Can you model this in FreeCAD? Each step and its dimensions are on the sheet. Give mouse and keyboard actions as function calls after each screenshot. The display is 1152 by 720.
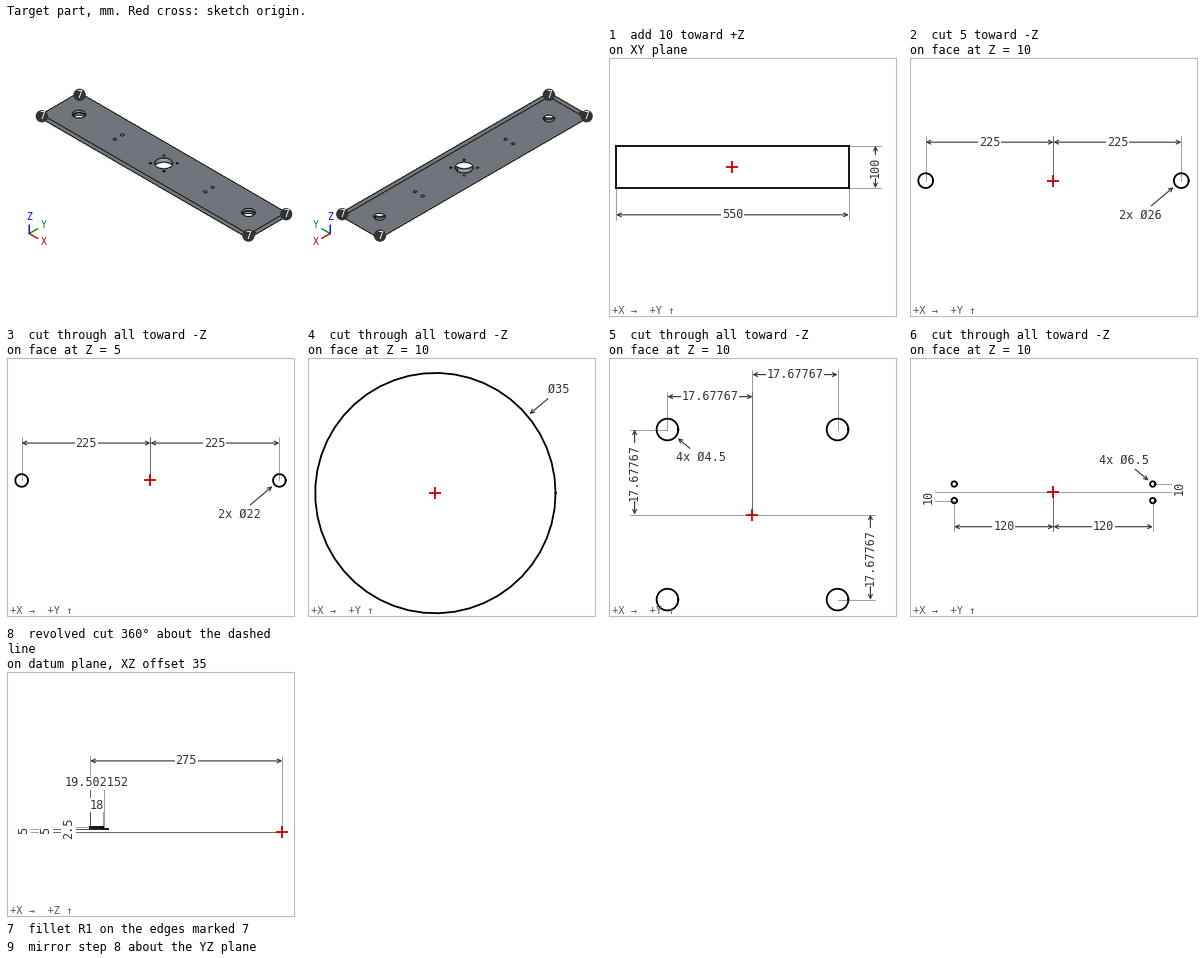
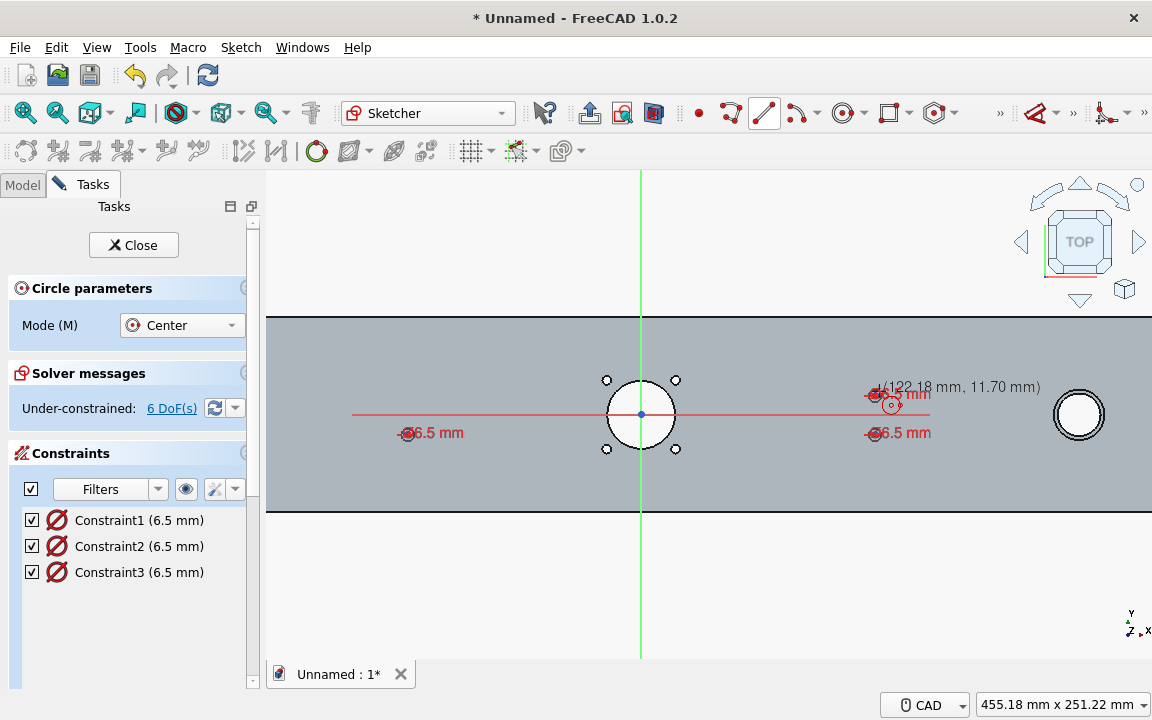
scroll(408, 395, up, 7)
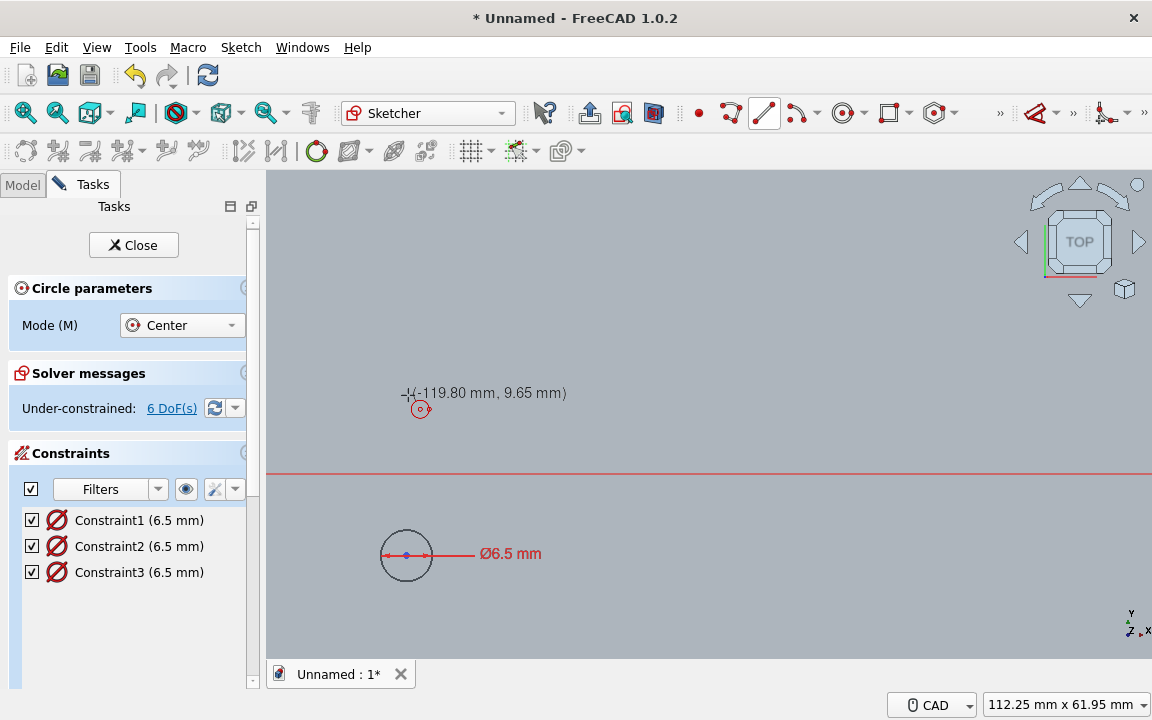
scroll(407, 395, down, 7)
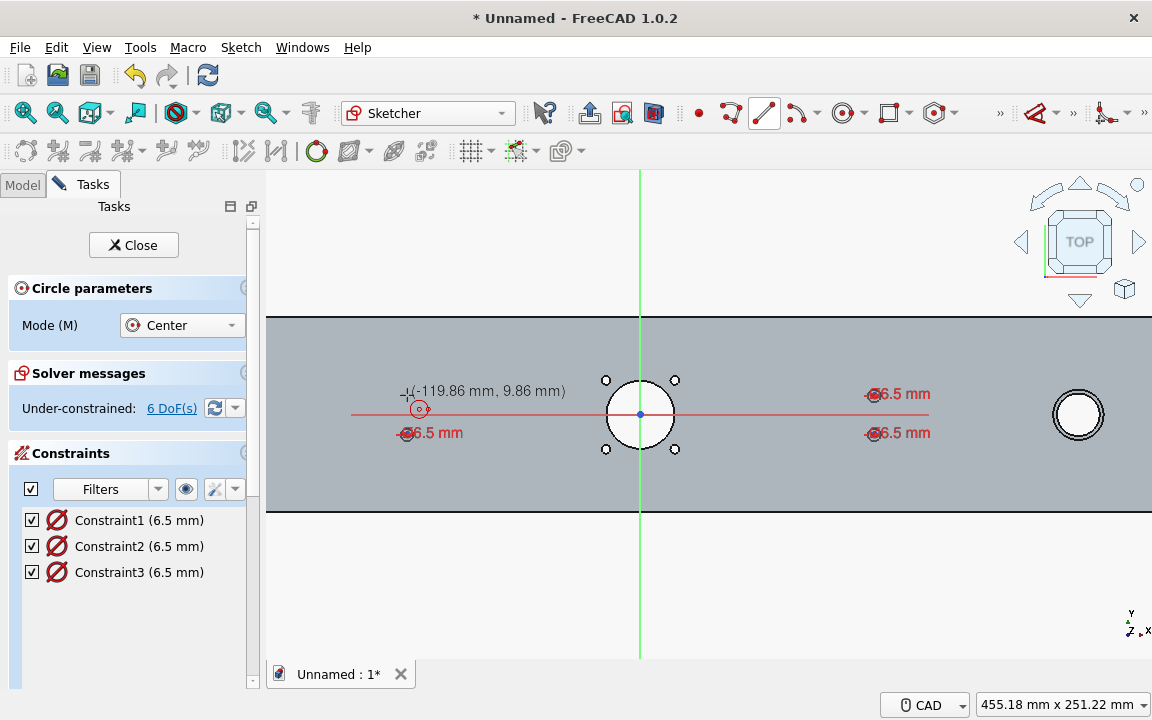
click(407, 395)
move(411, 391)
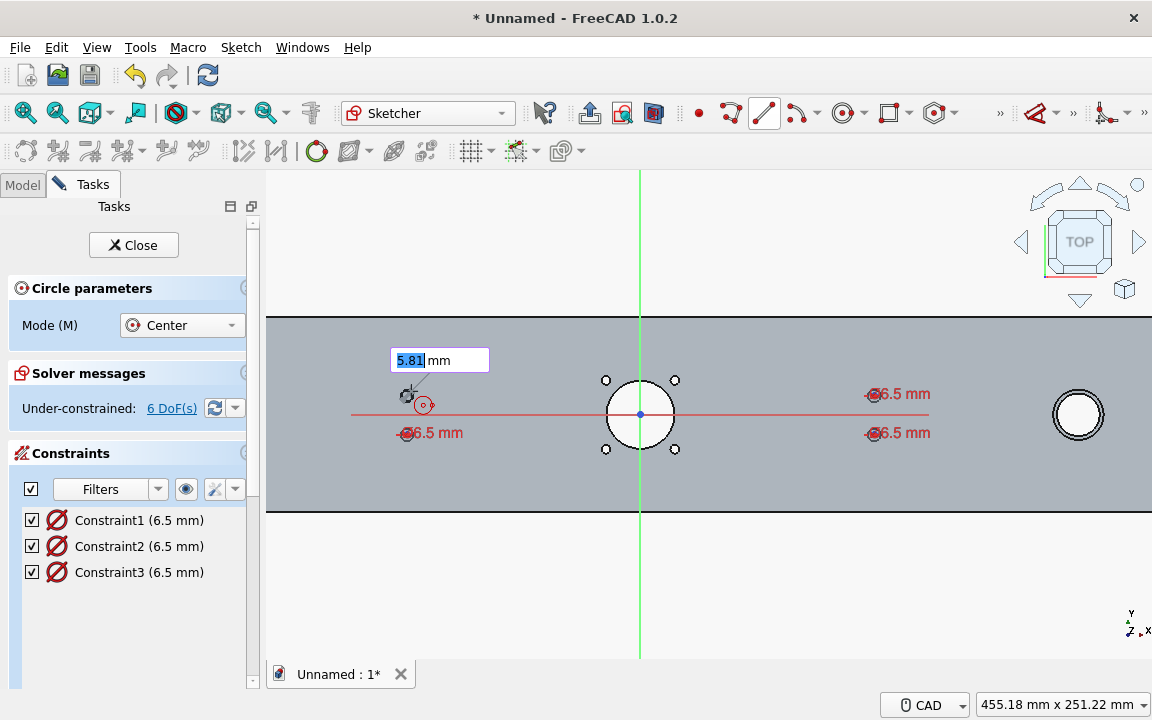
text(6.5)
key(Return)
key(Escape)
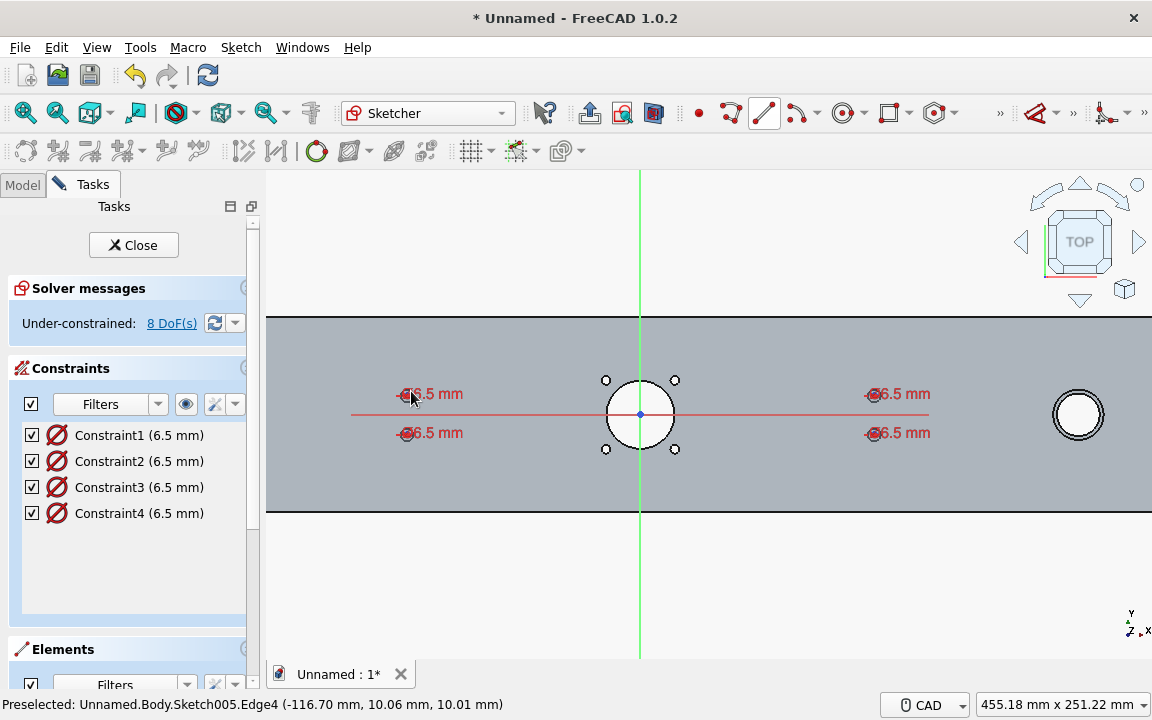
click(407, 435)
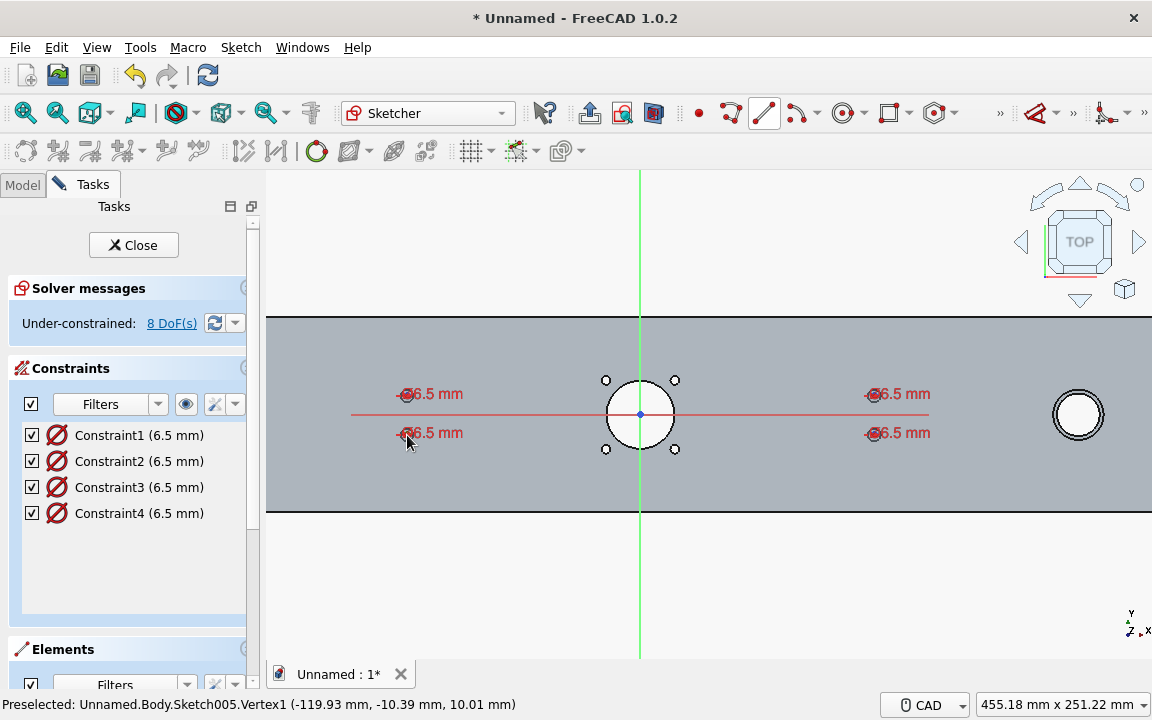
click(874, 435)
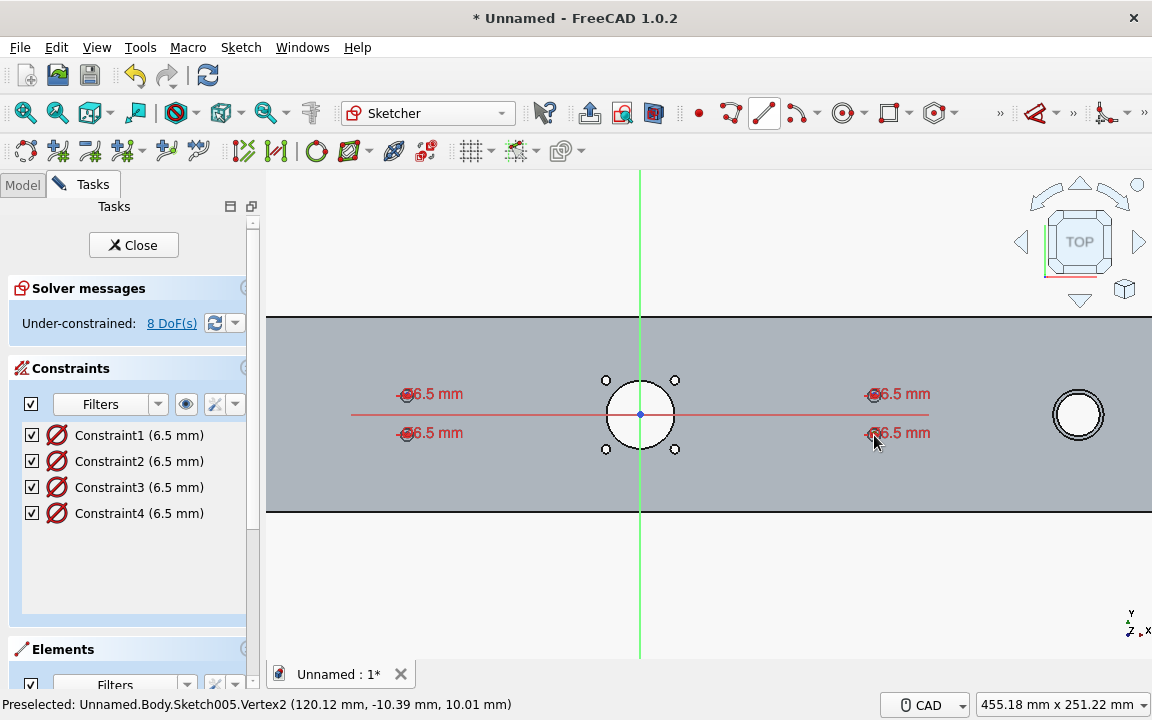
key(h)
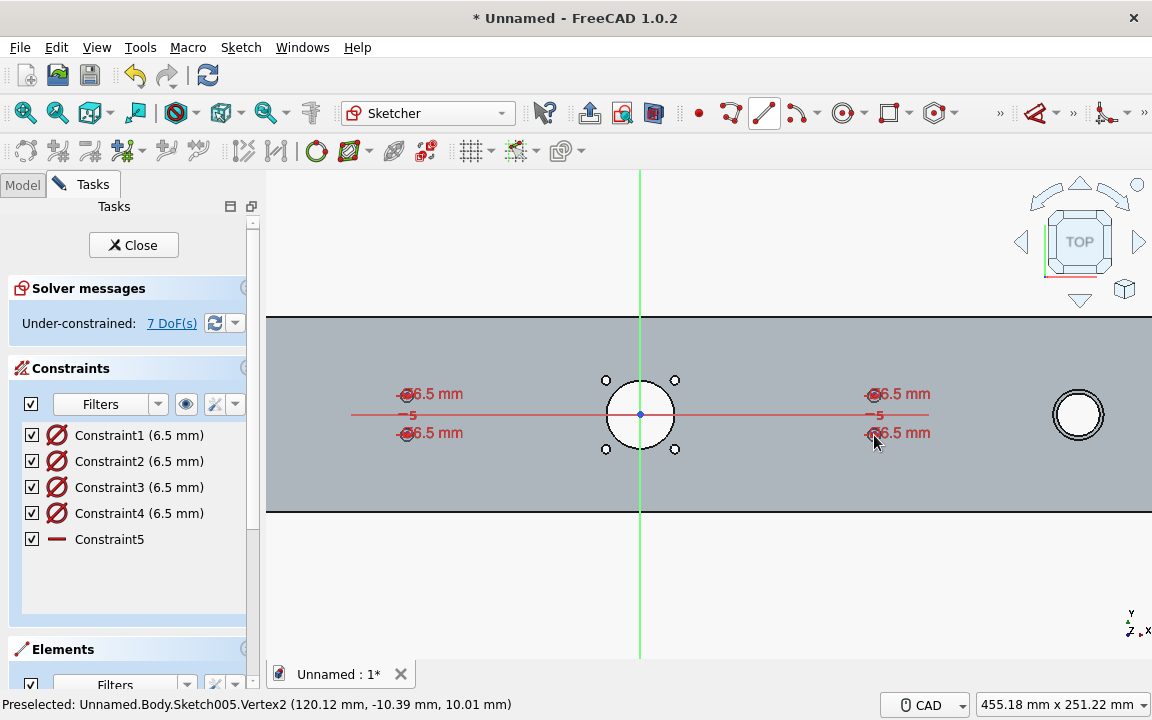
click(874, 435)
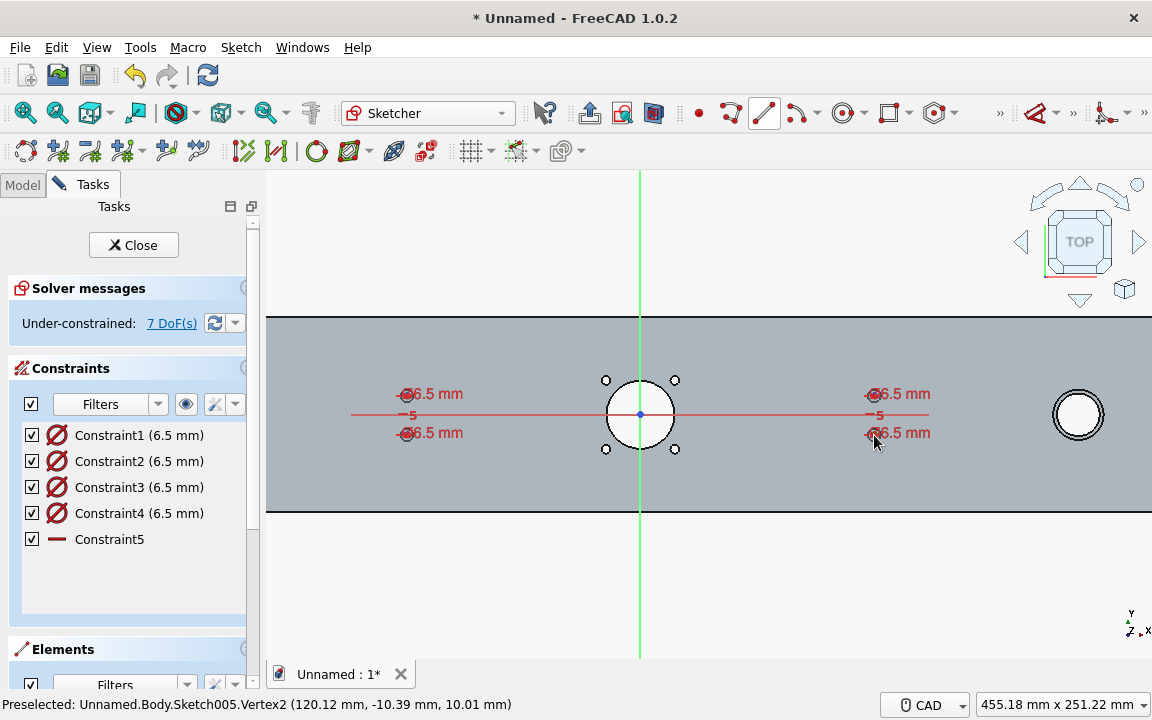
click(874, 396)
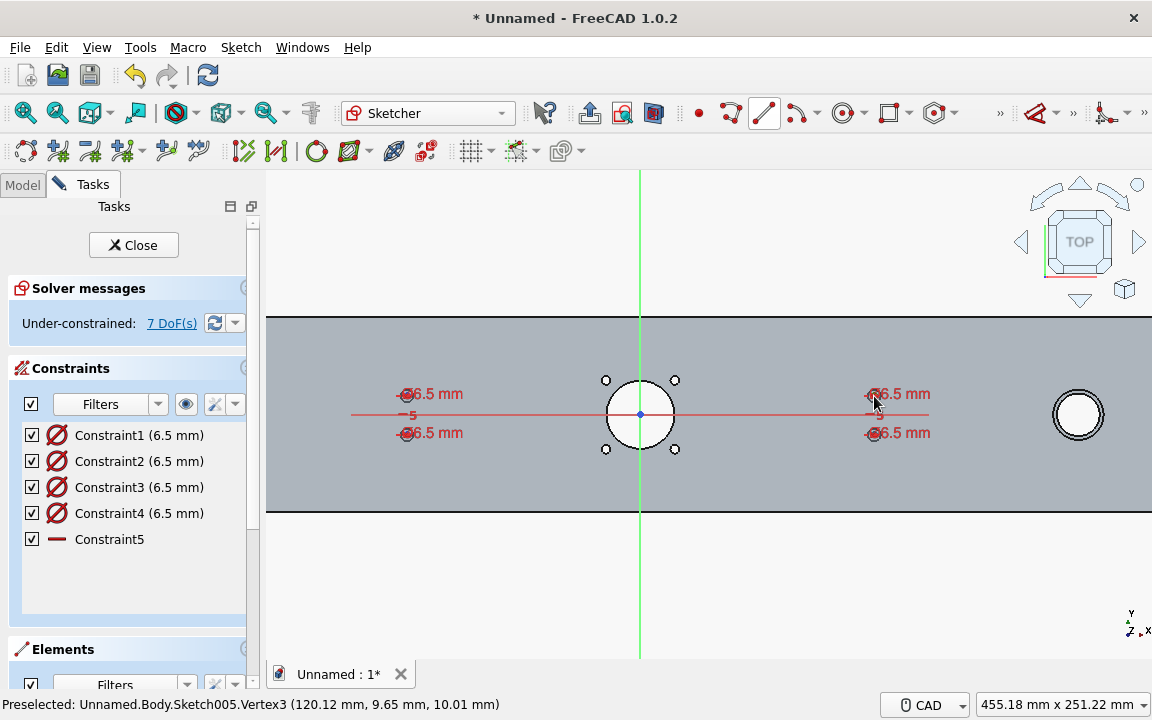
key(v)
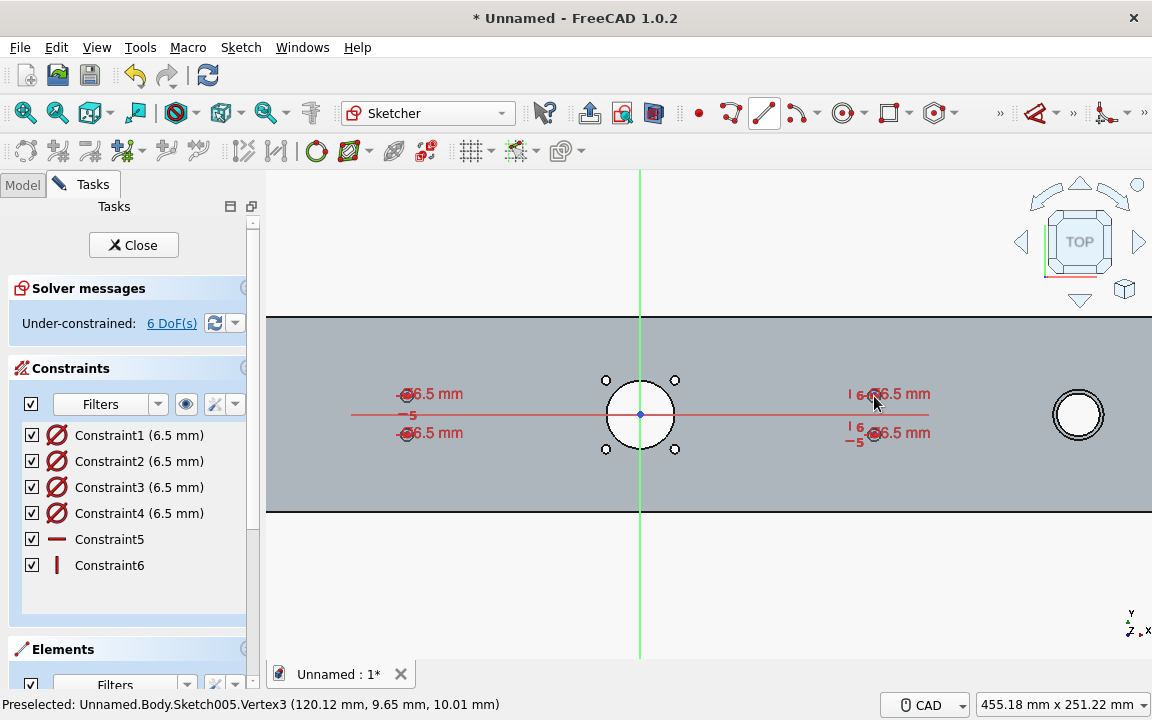
click(407, 435)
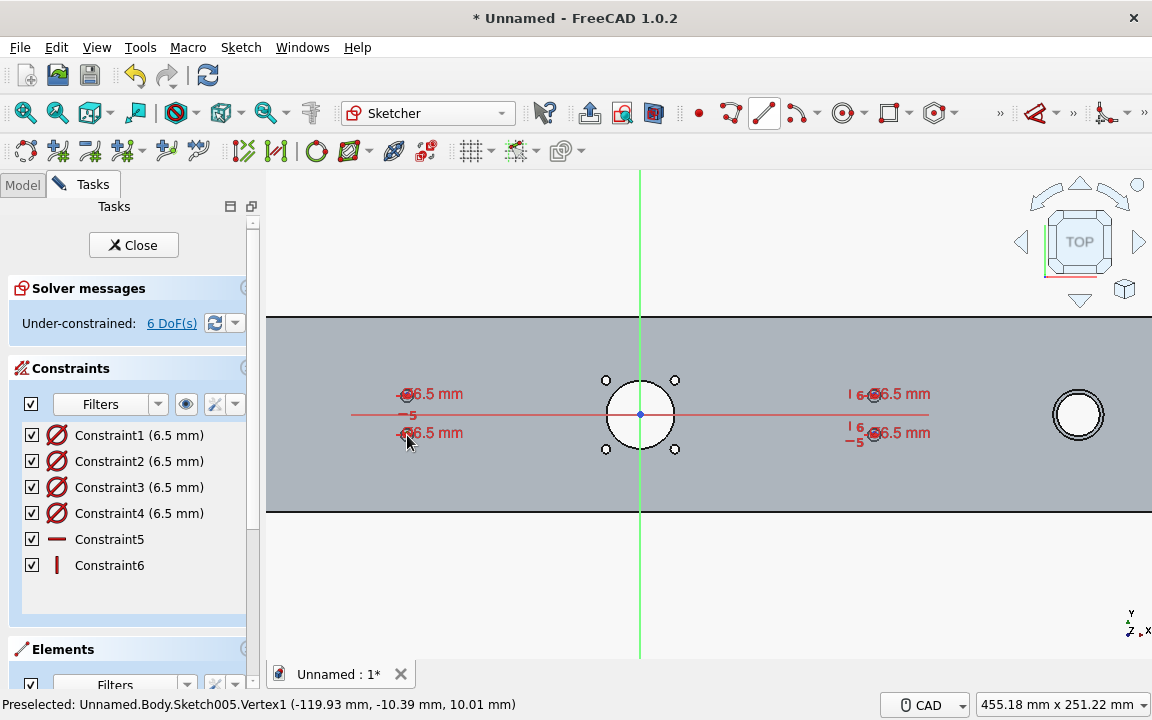
click(407, 396)